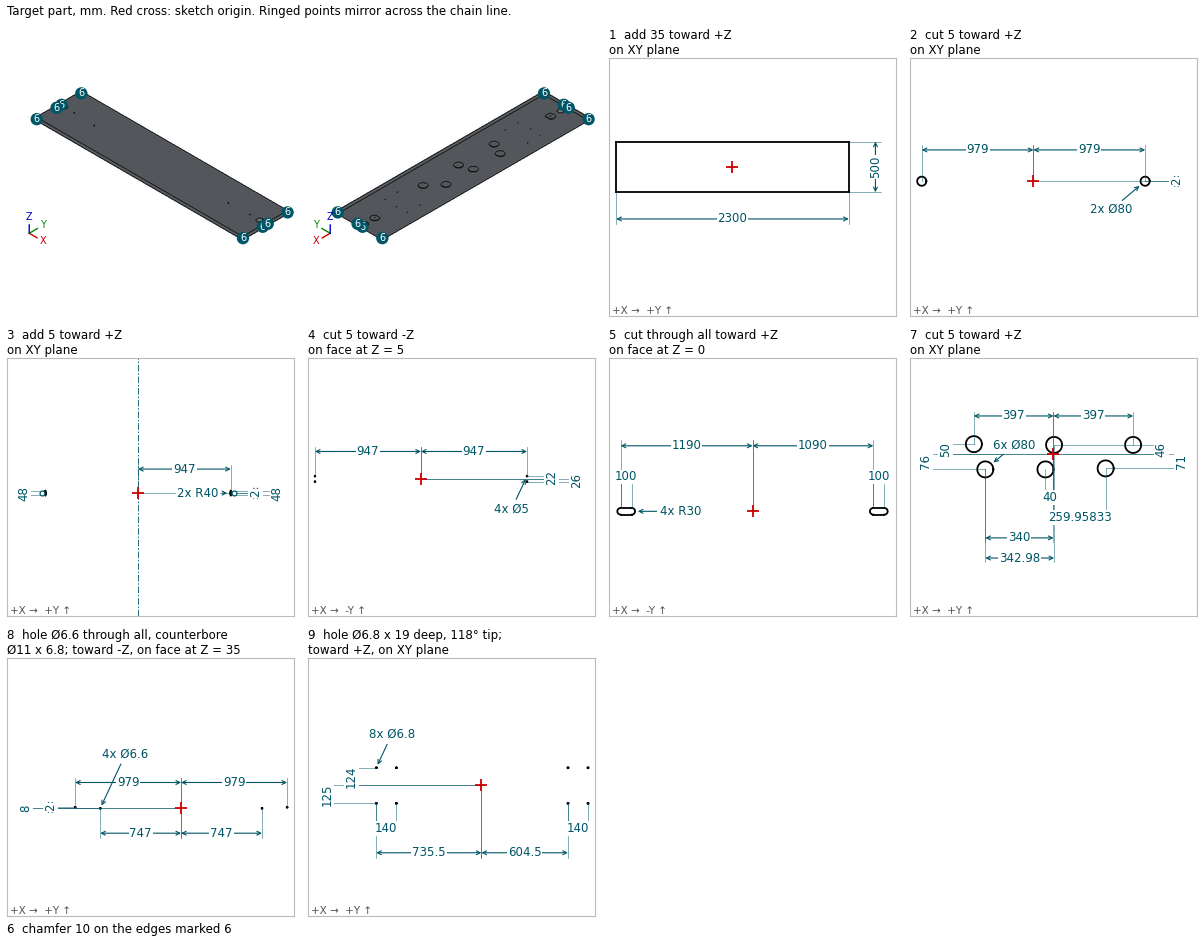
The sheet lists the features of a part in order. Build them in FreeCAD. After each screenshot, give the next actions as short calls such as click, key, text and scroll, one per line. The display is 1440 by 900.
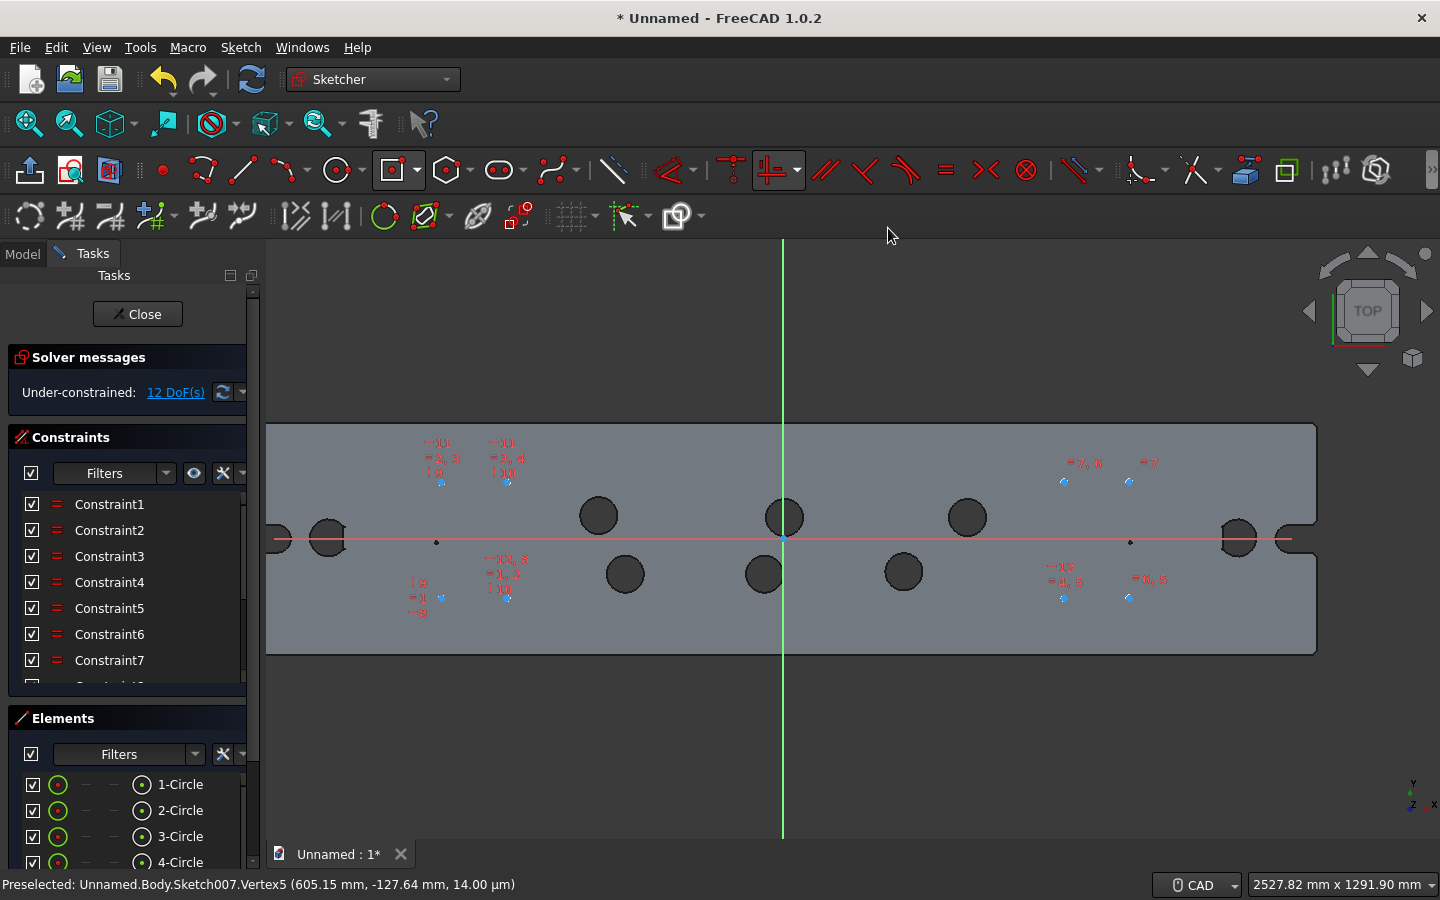
click(1064, 598)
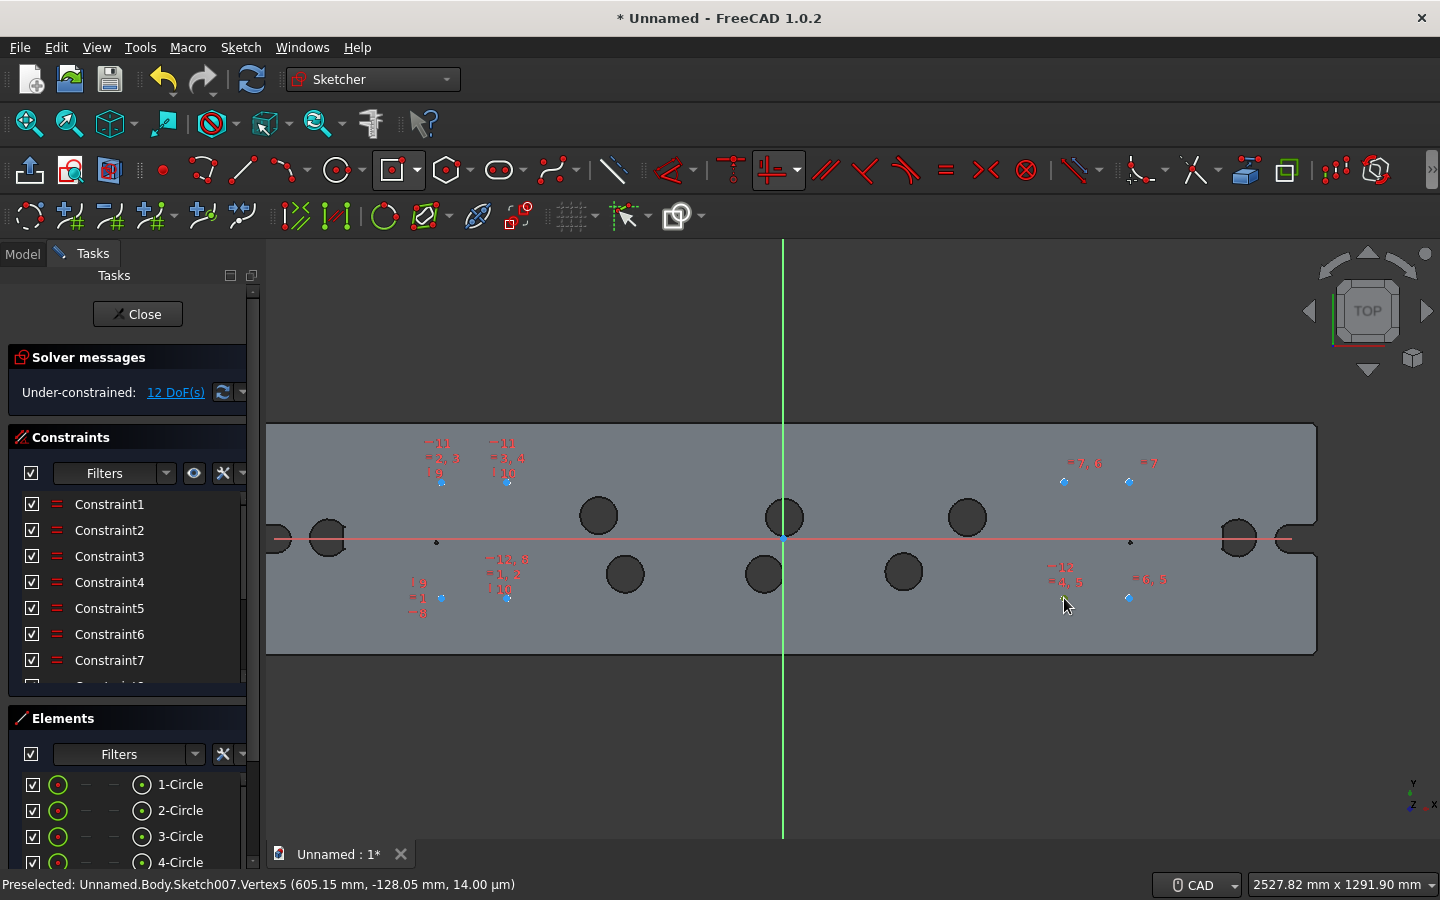
click(1129, 598)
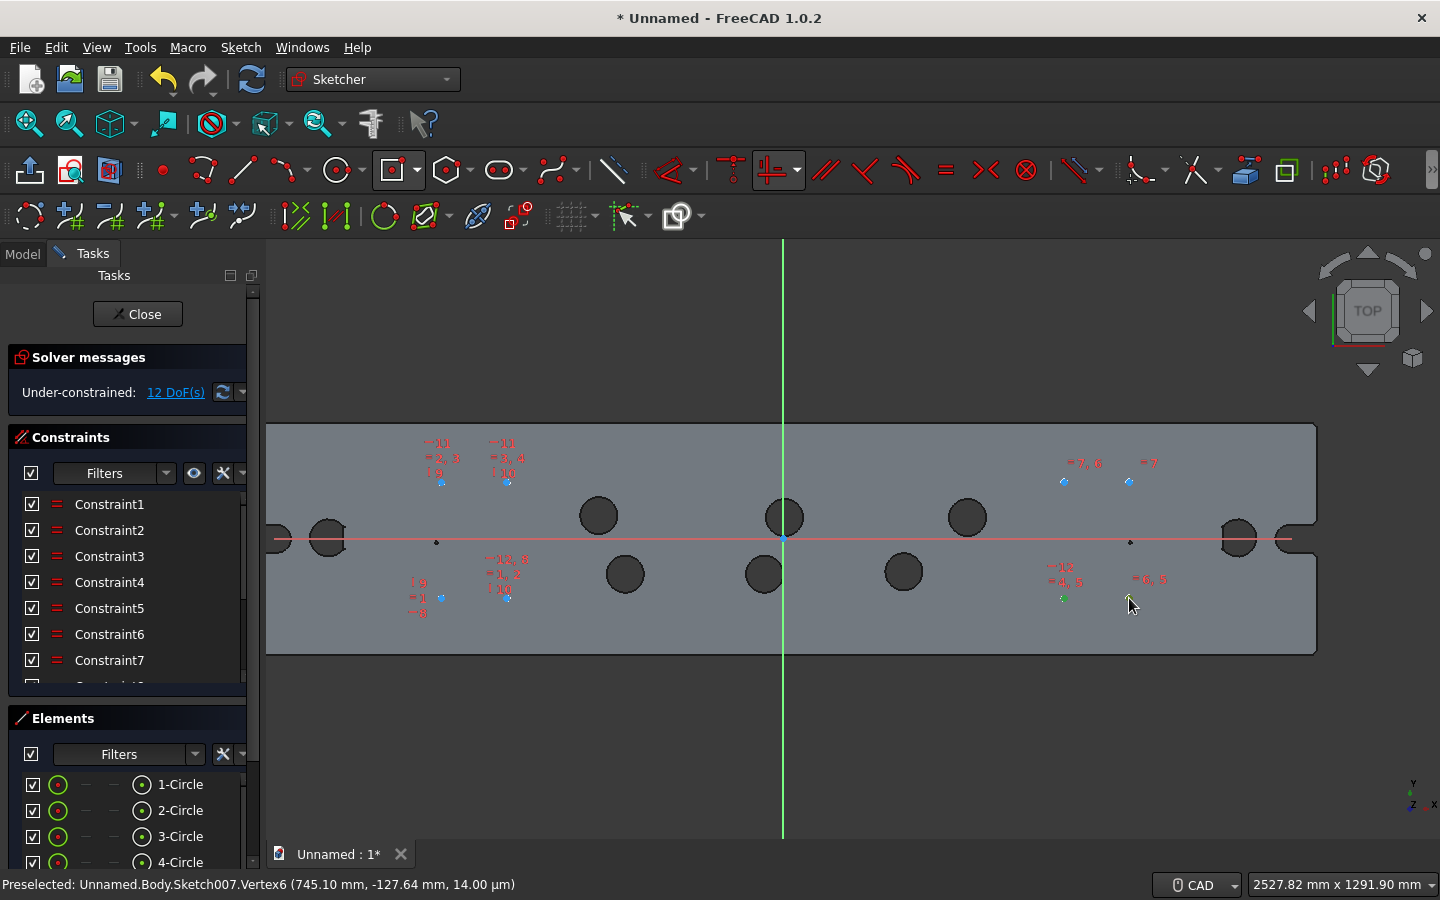
key(h)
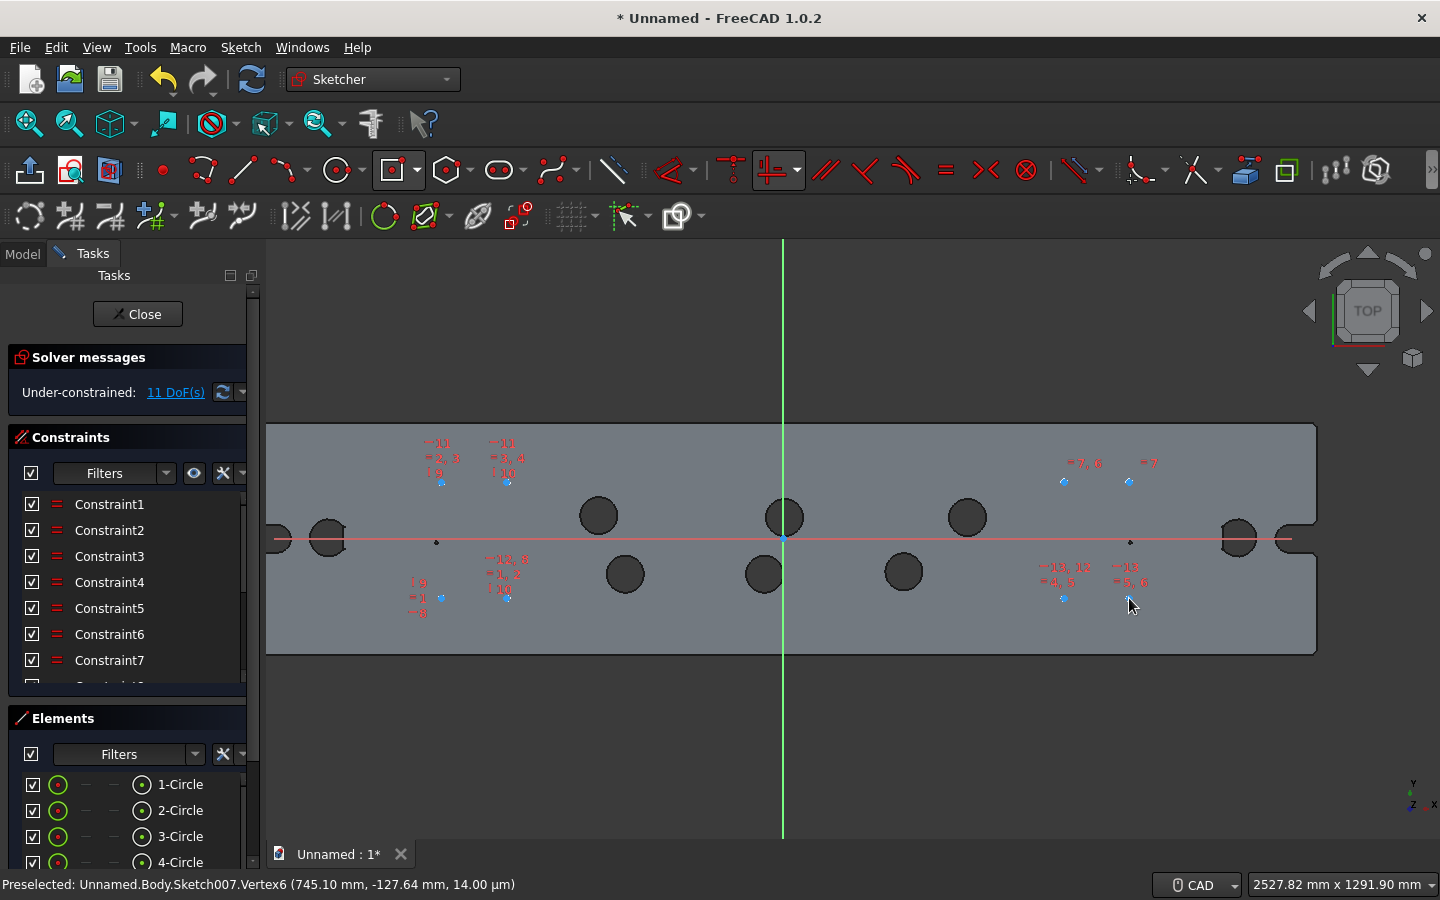
click(1064, 598)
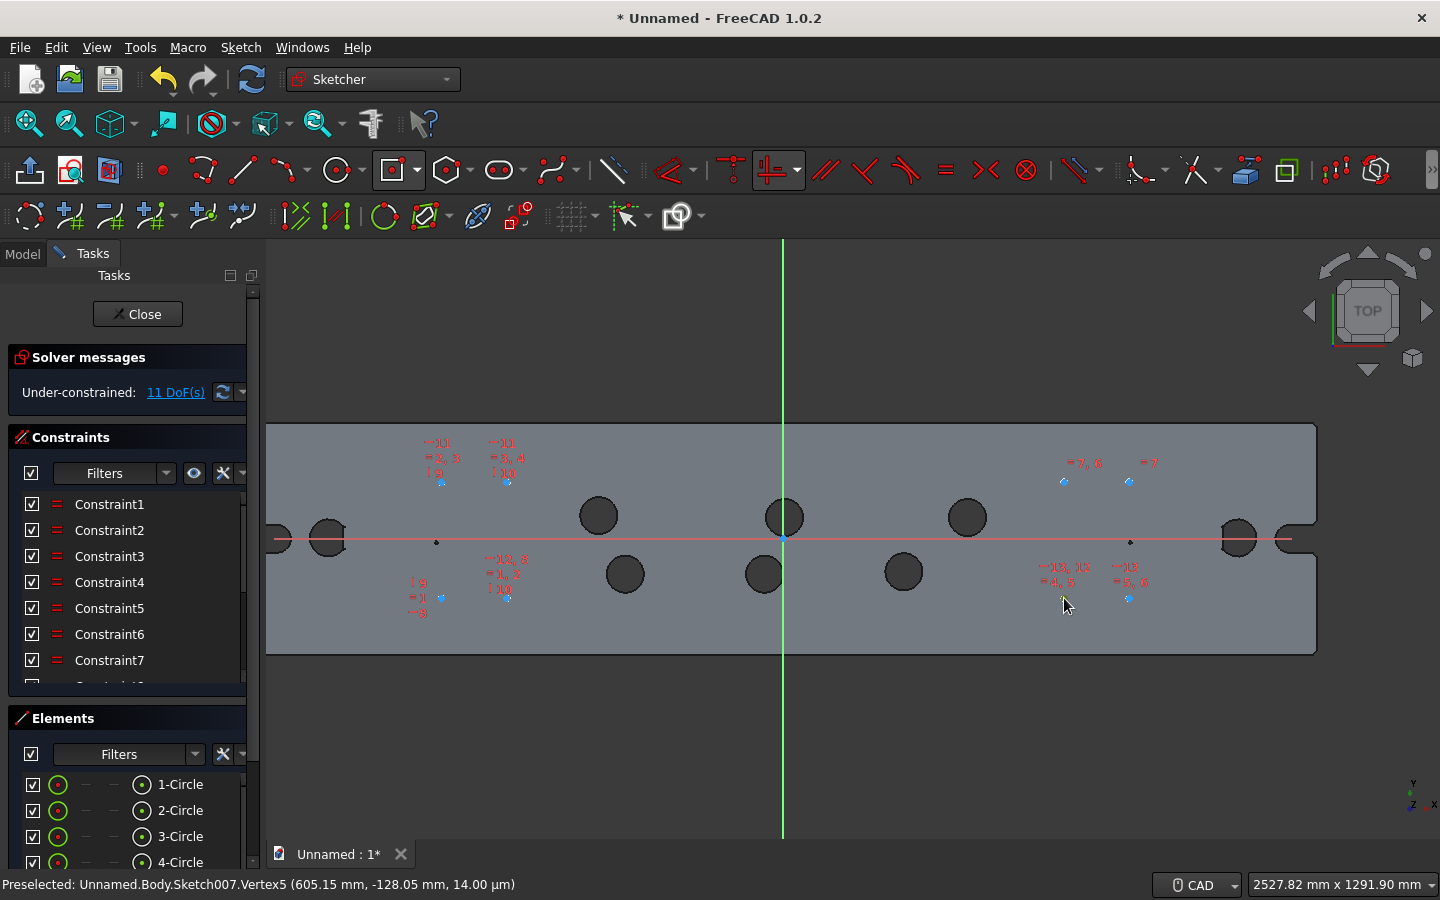
click(1064, 482)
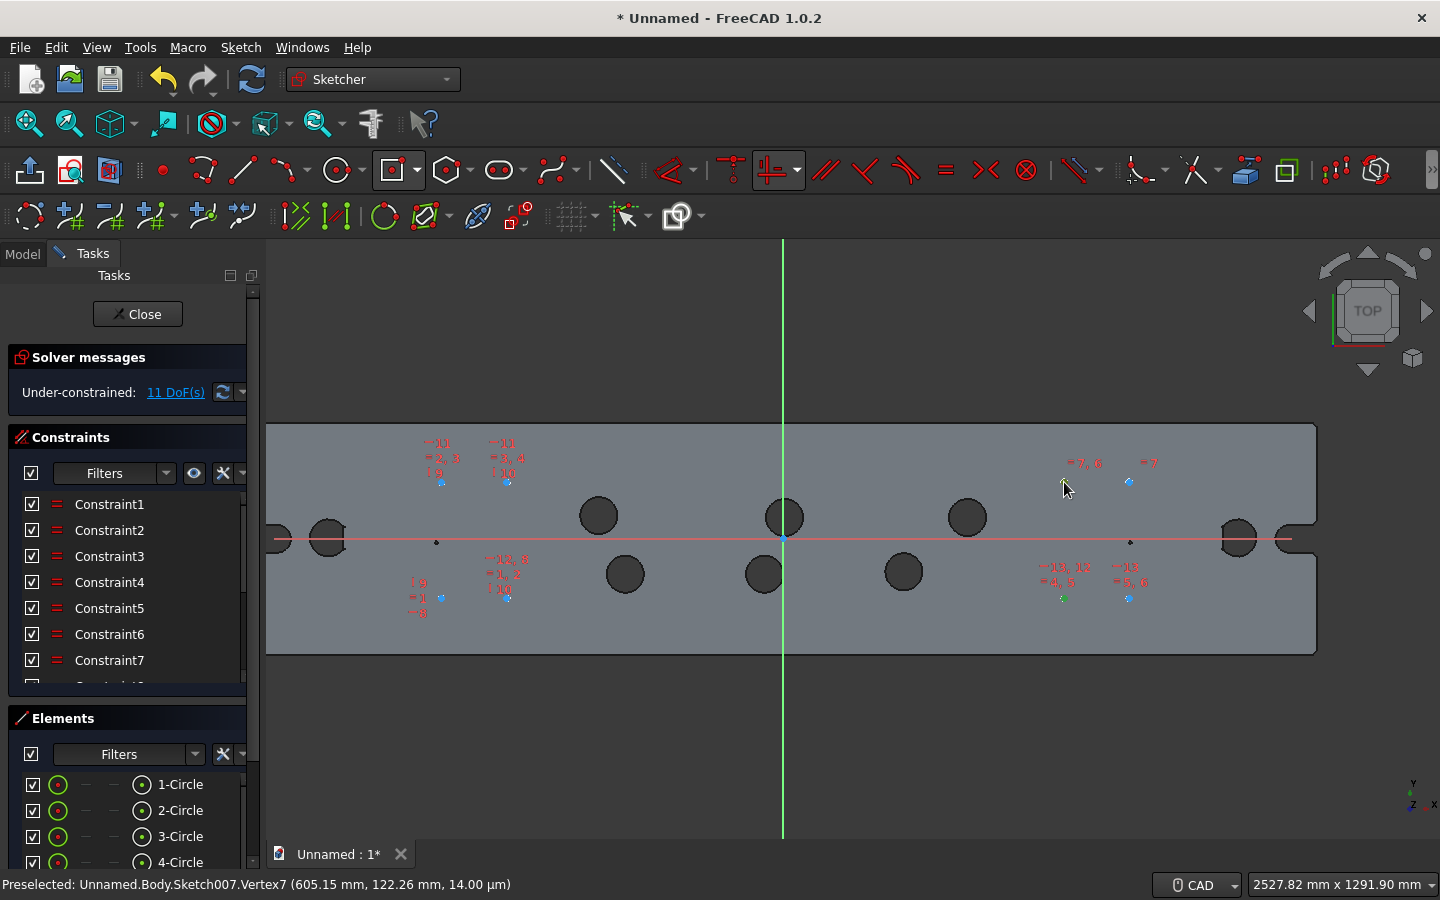
click(800, 170)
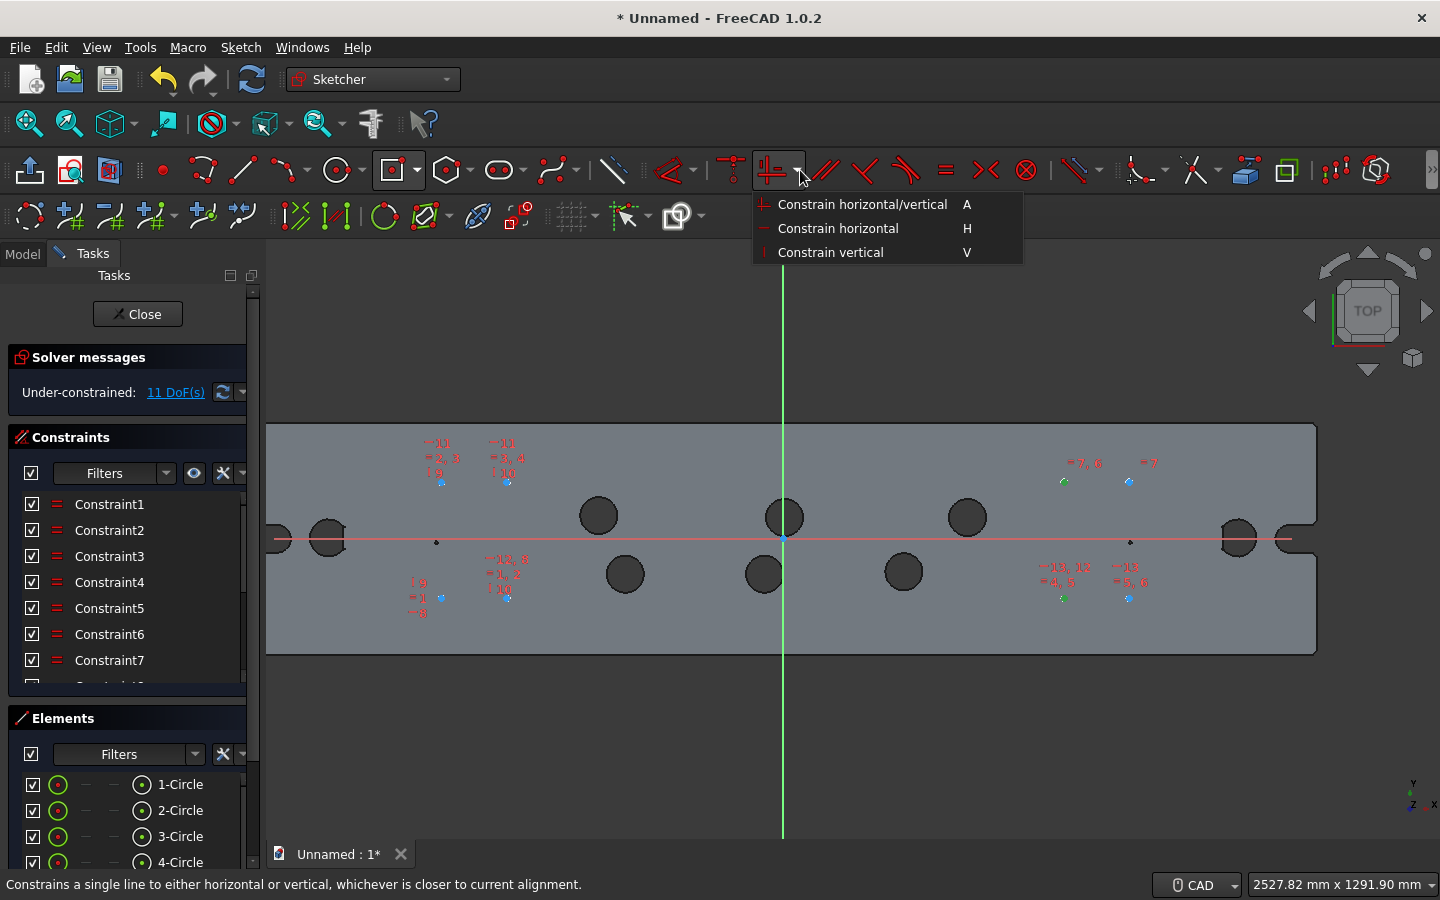
click(888, 252)